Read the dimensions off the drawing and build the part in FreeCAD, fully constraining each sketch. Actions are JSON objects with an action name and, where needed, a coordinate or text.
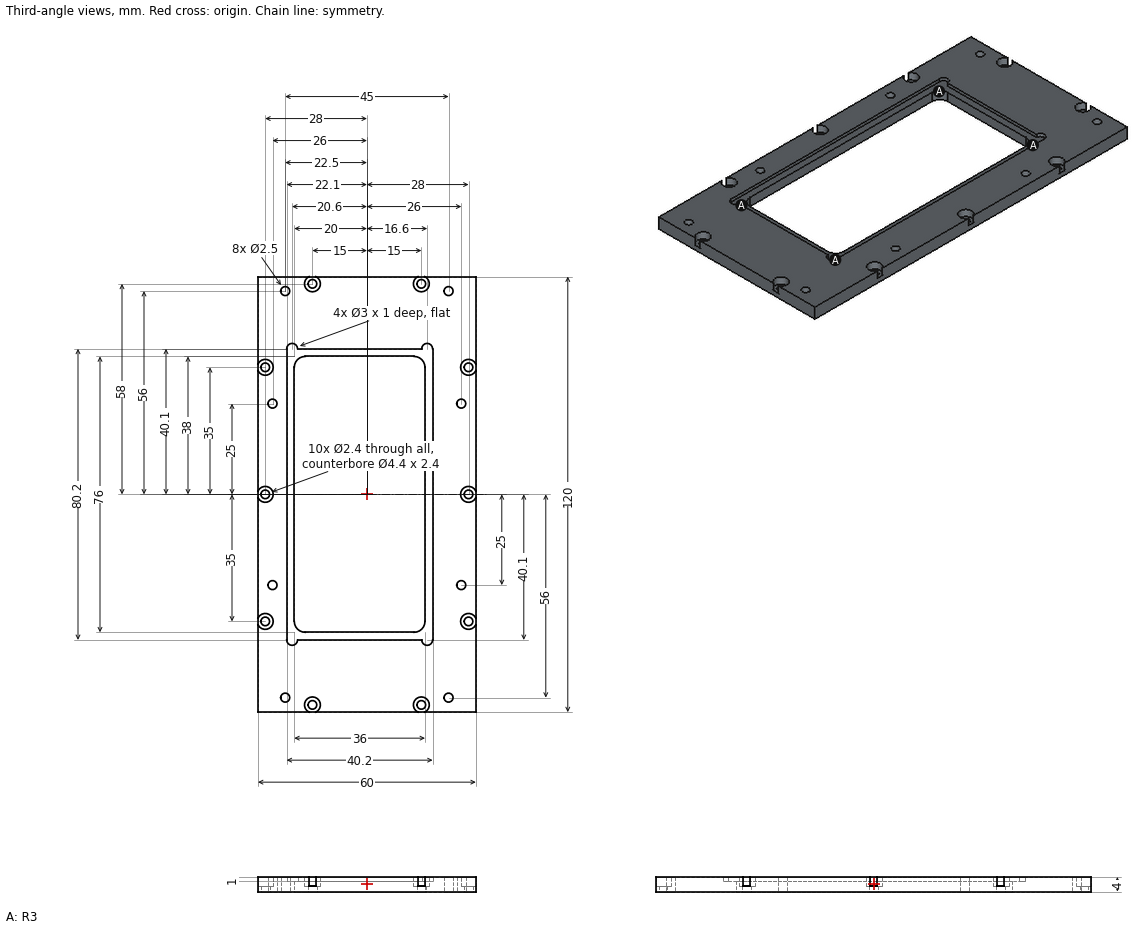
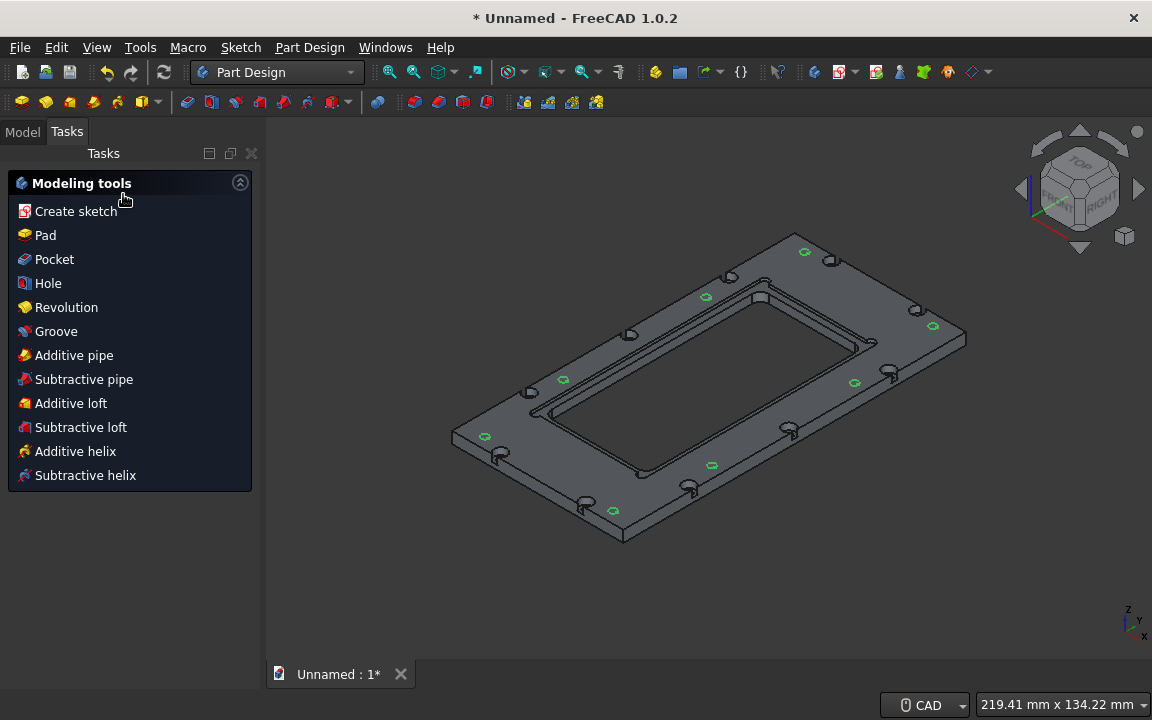
{"action": "left_click", "coordinate": [188, 102]}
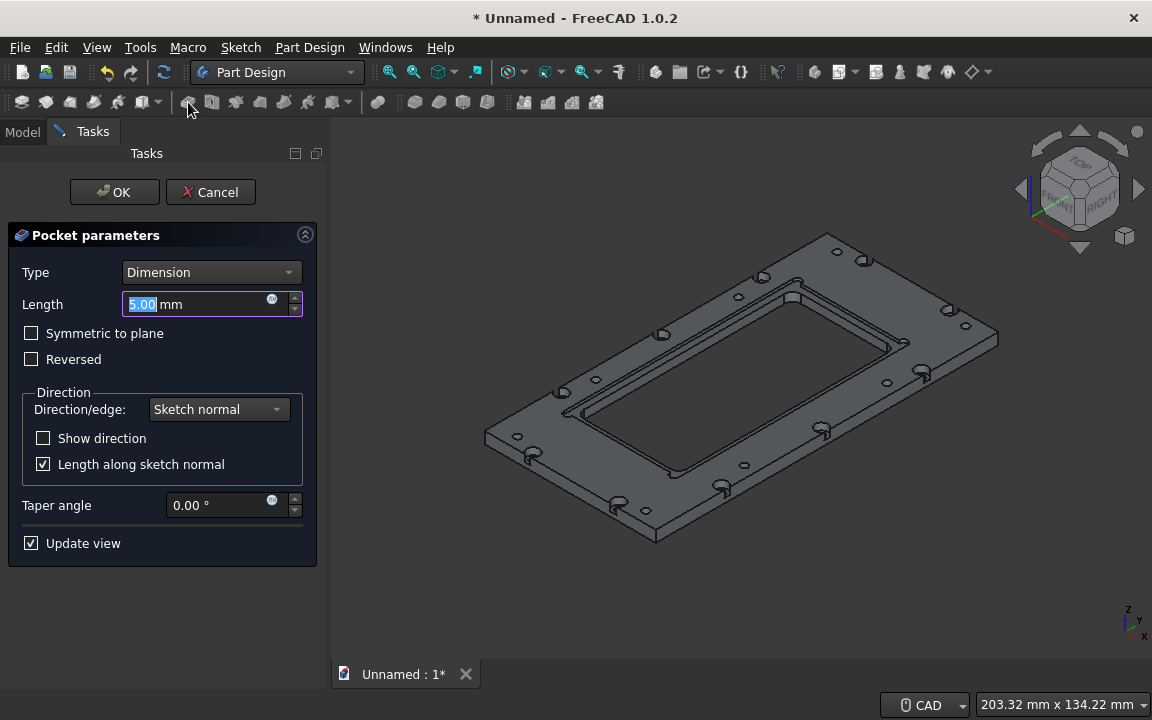
{"action": "left_click", "coordinate": [212, 272]}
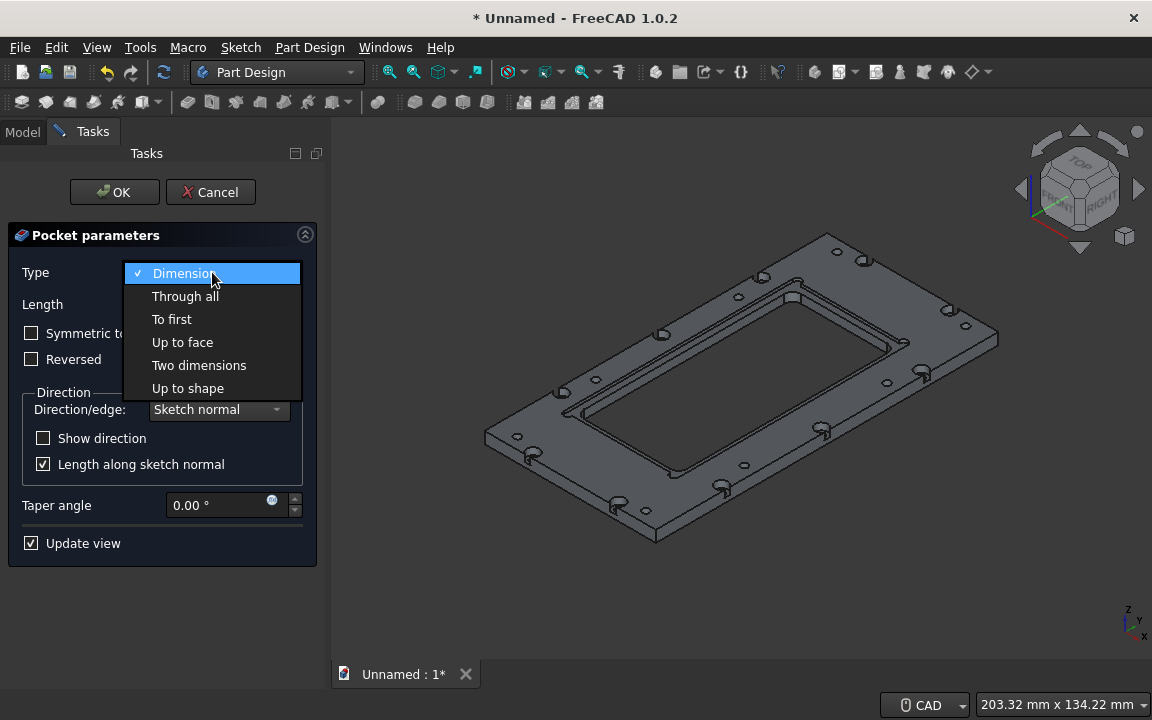
{"action": "left_click", "coordinate": [212, 296]}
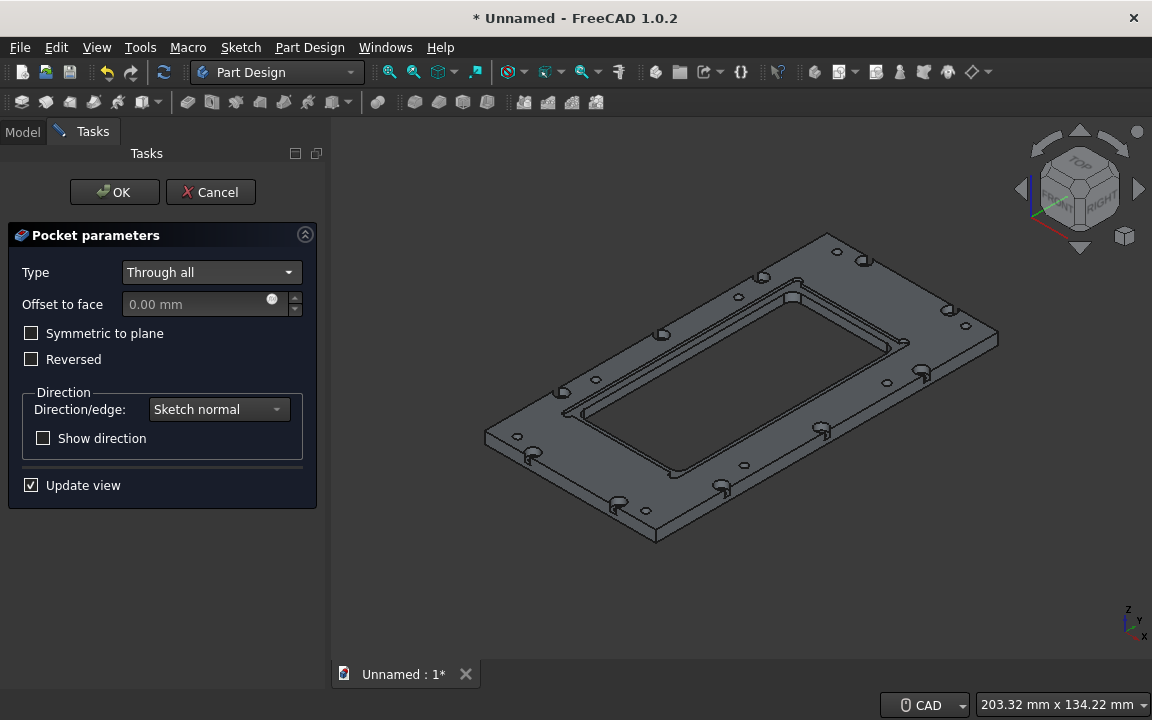
{"action": "left_click", "coordinate": [115, 192]}